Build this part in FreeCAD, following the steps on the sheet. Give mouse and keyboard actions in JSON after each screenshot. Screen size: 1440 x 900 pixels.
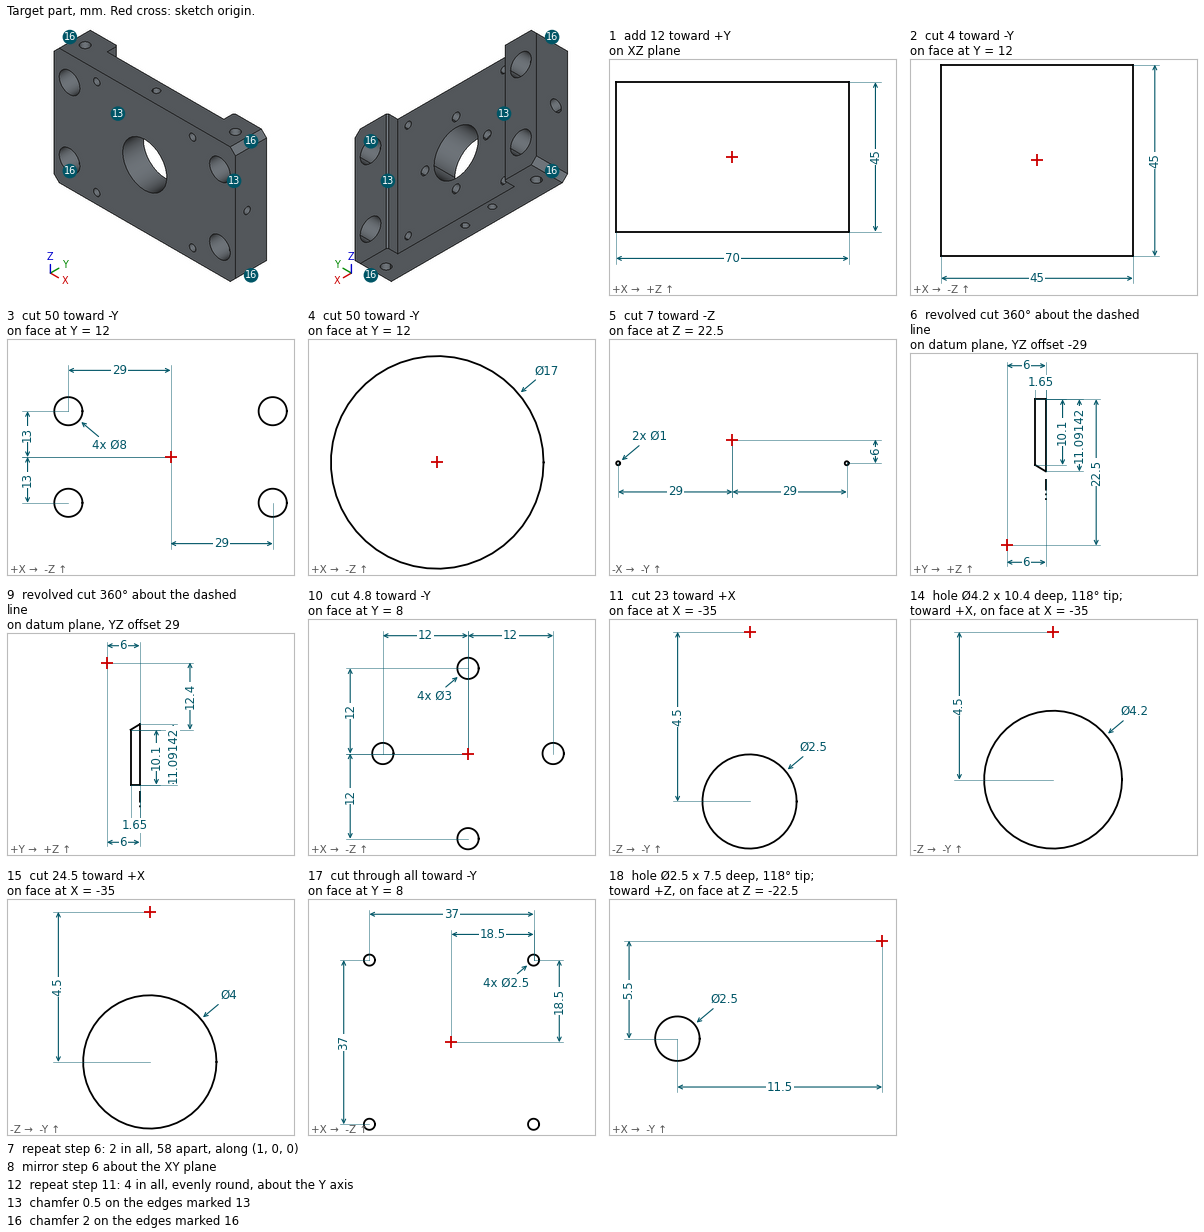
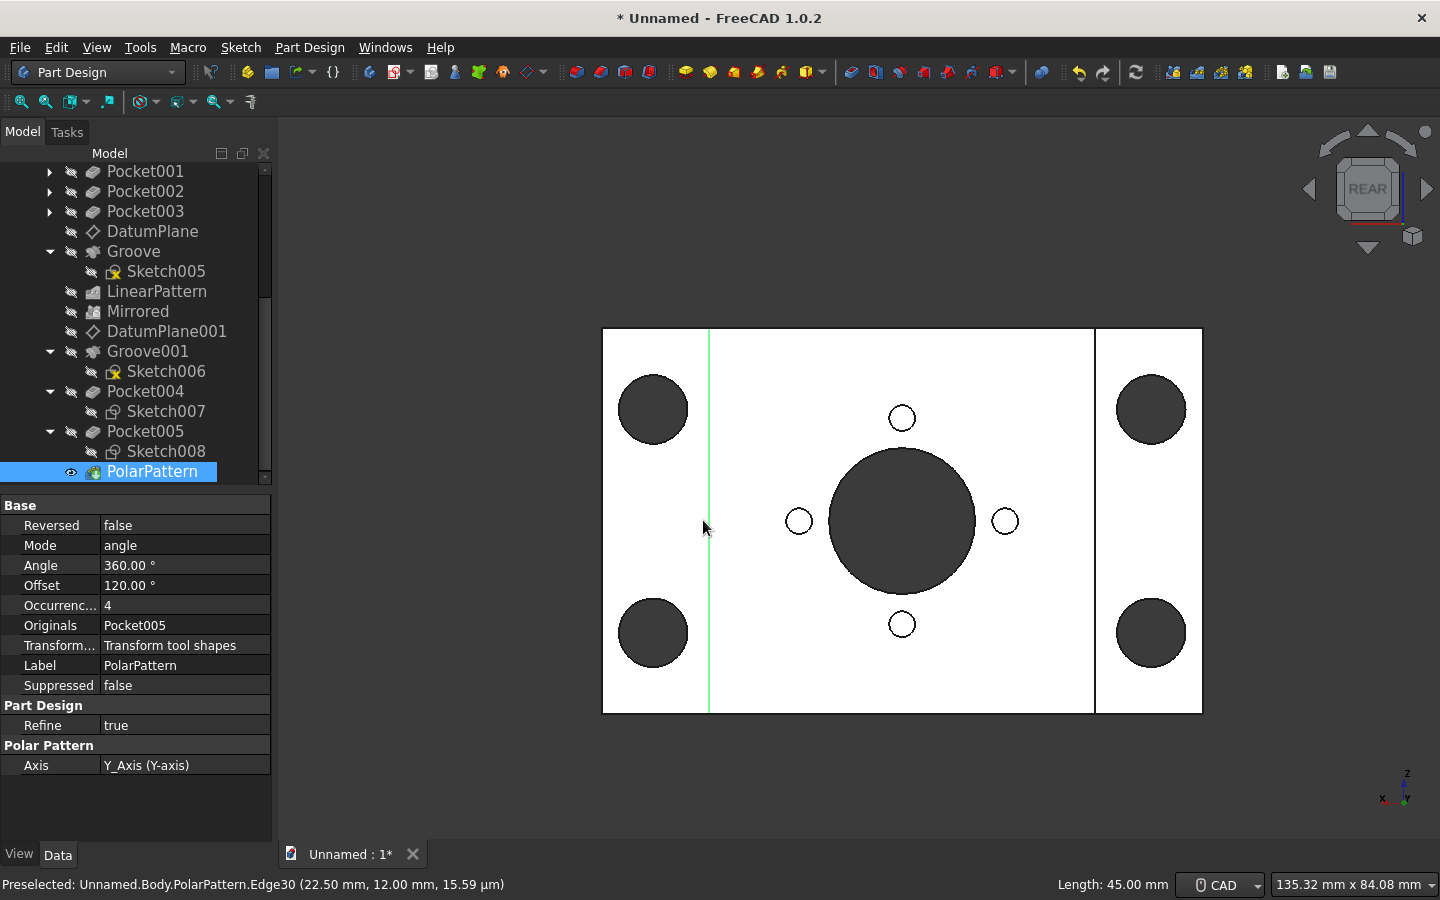
{"action": "left_click", "coordinate": [1095, 520], "text": "ctrl"}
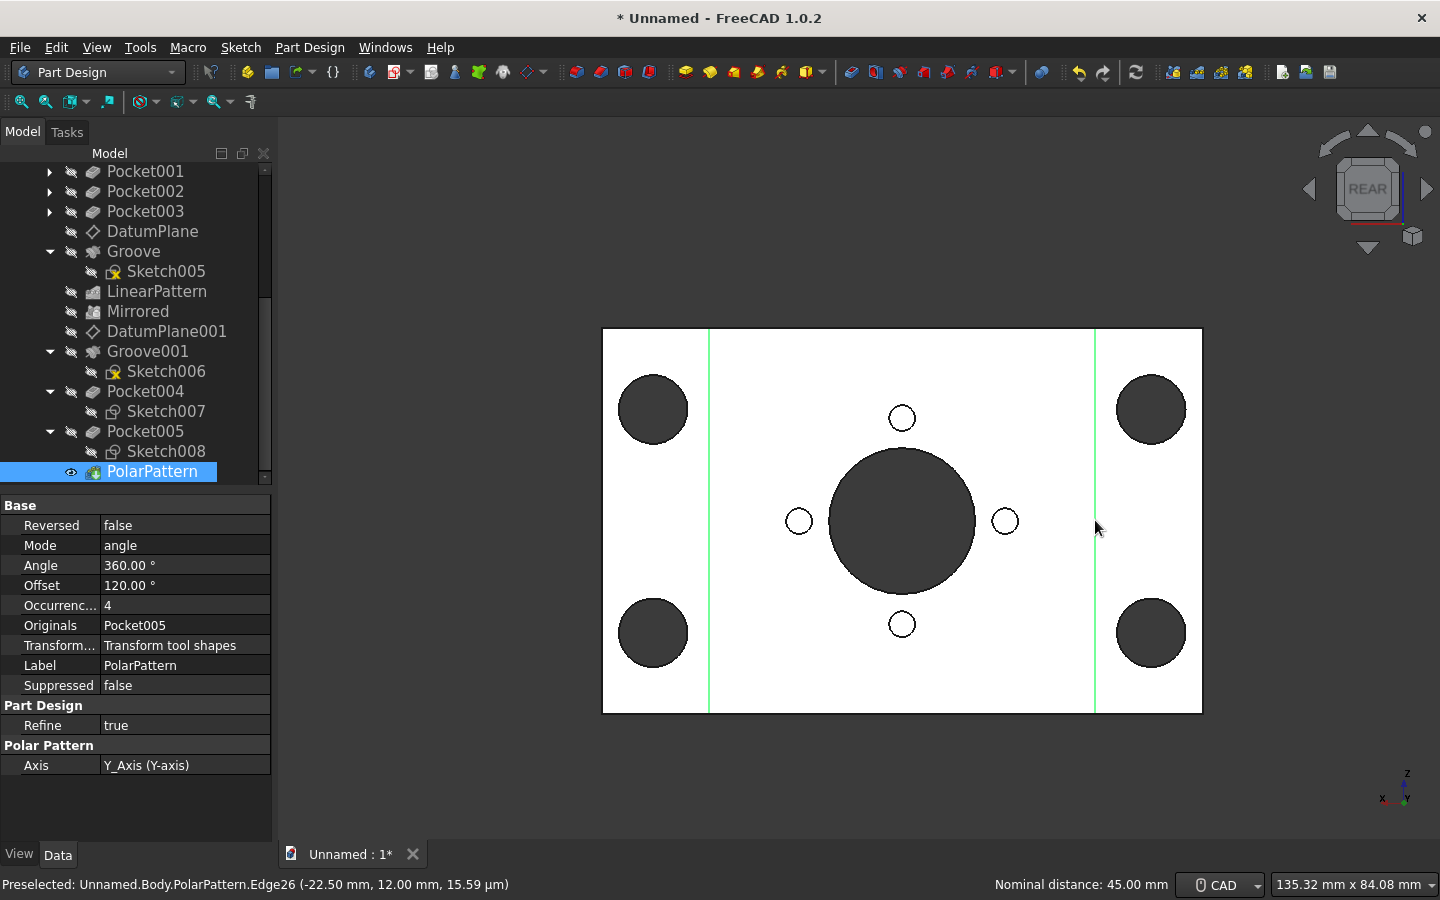
{"action": "left_click", "coordinate": [602, 72]}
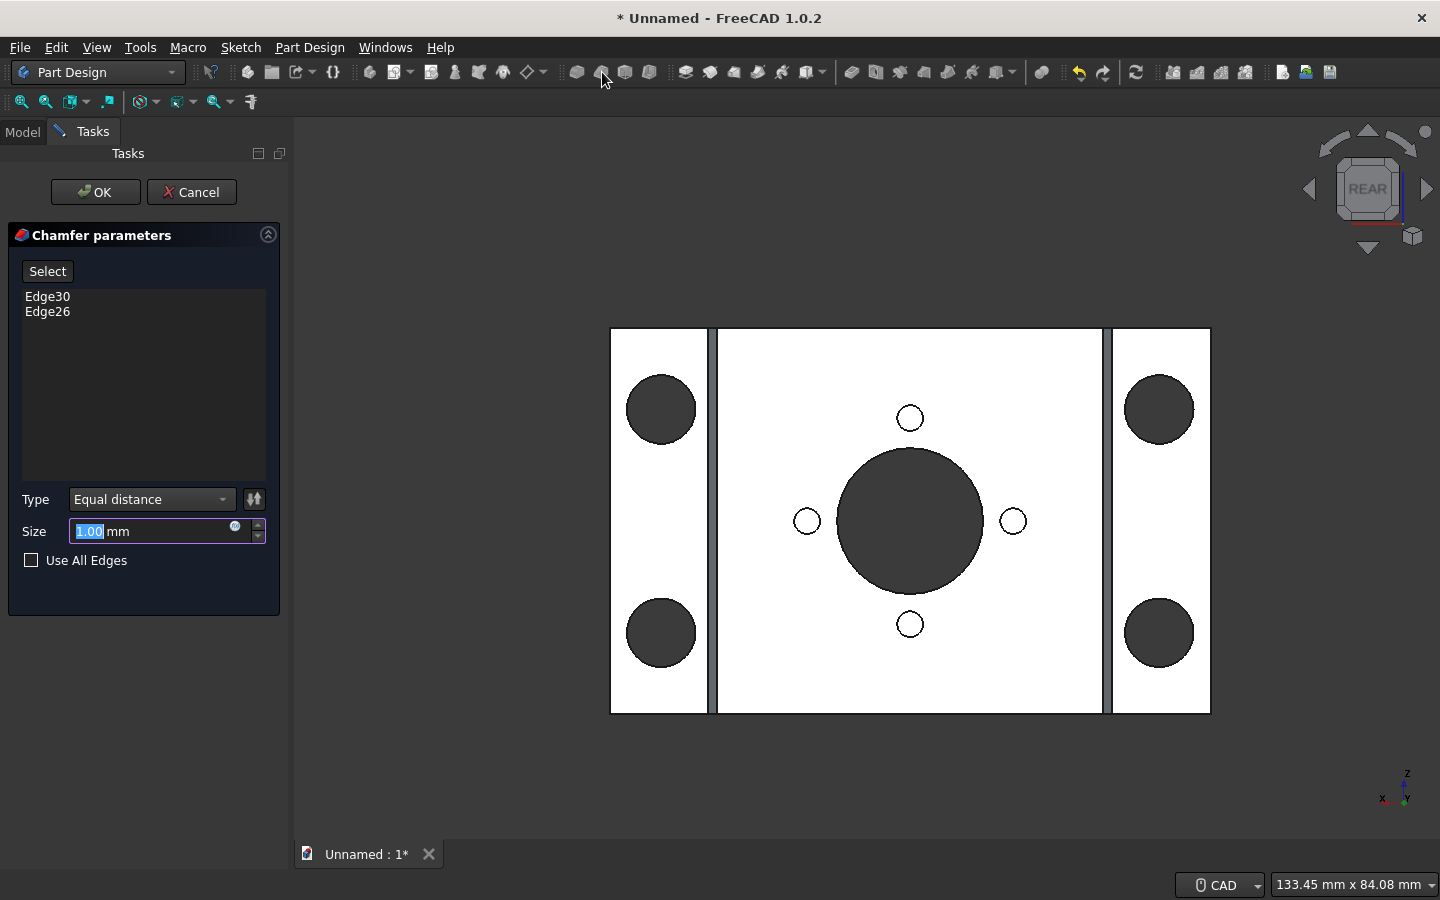
{"action": "type", "text": "0.5"}
{"action": "key", "text": "Tab"}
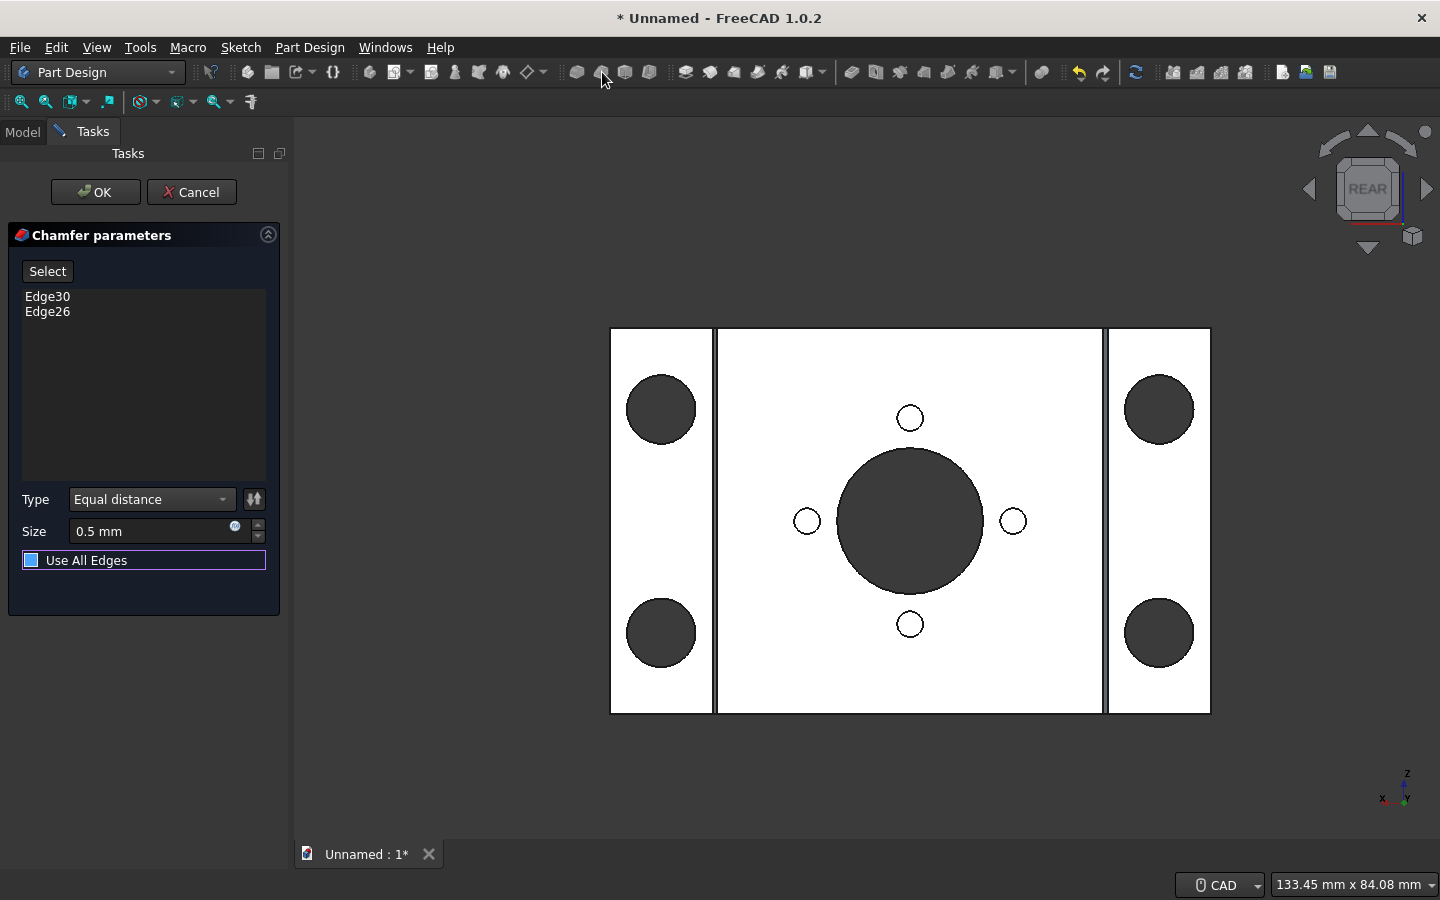
{"action": "left_click", "coordinate": [96, 192]}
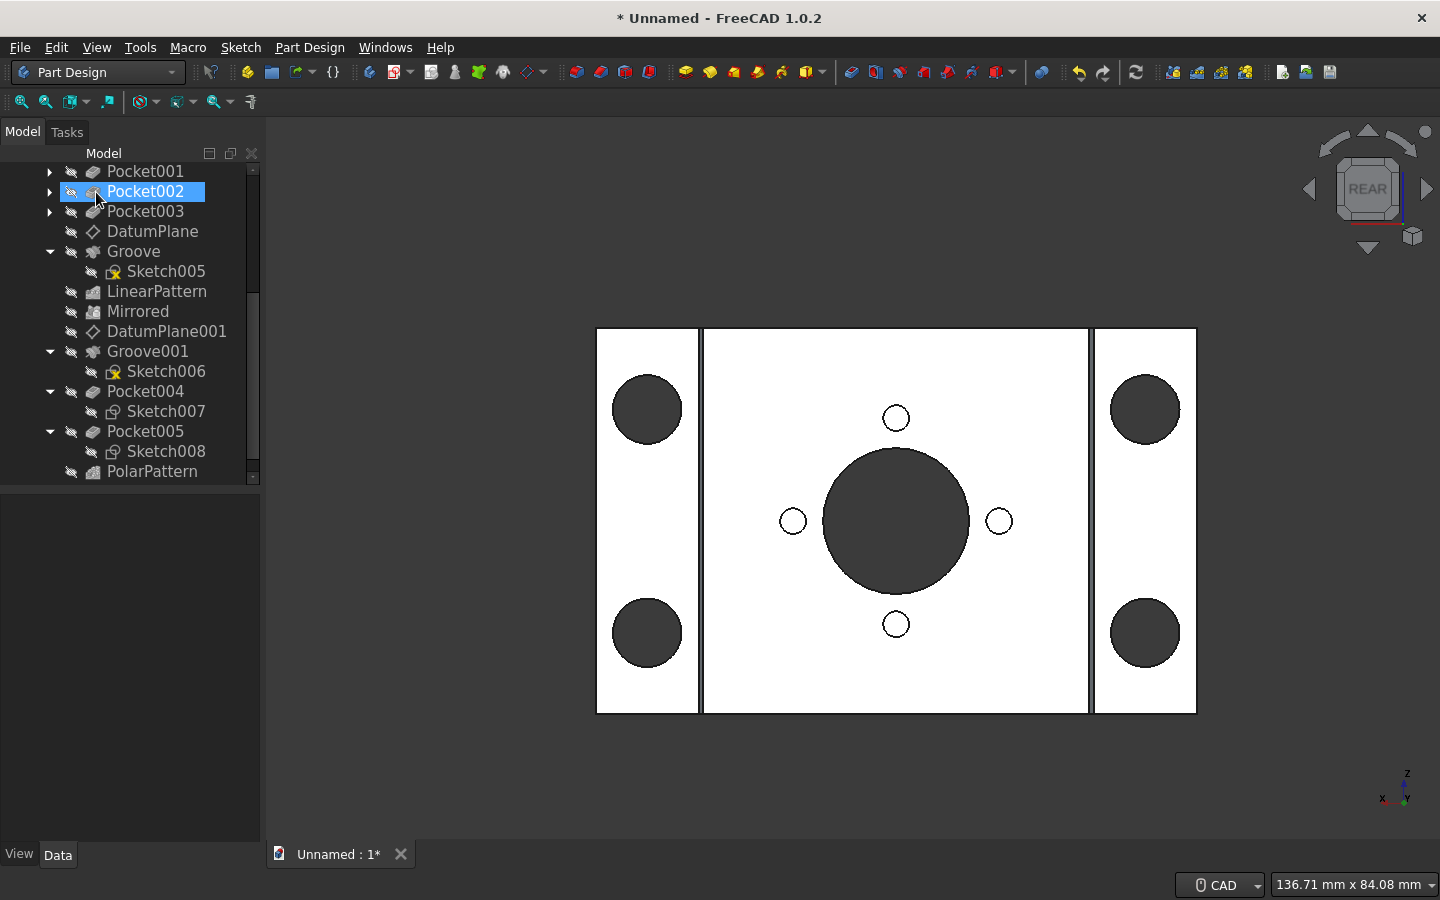
{"action": "key", "text": "6"}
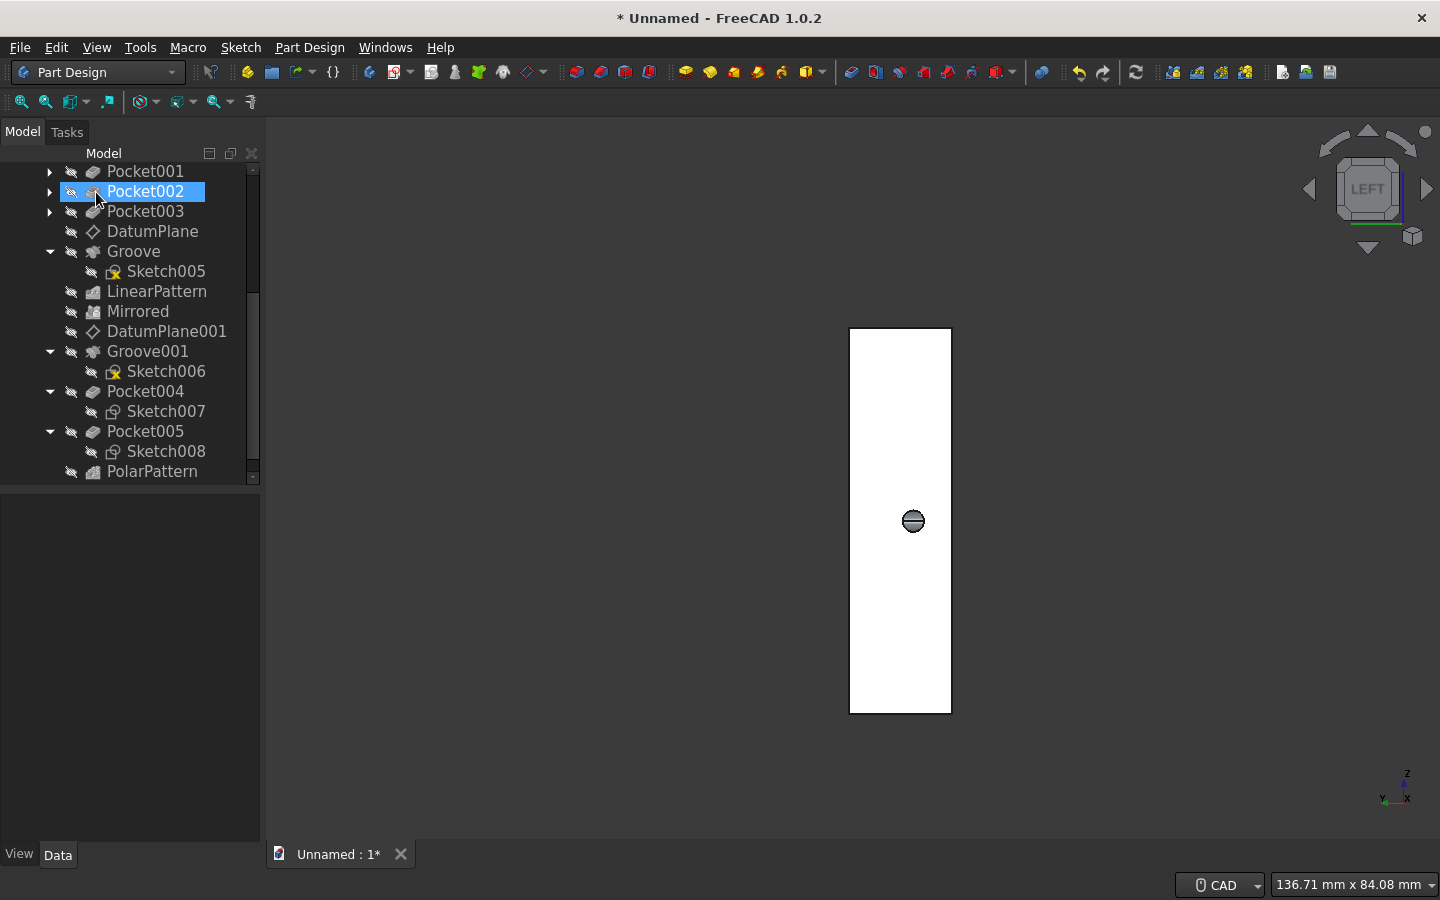
{"action": "left_click", "coordinate": [900, 410]}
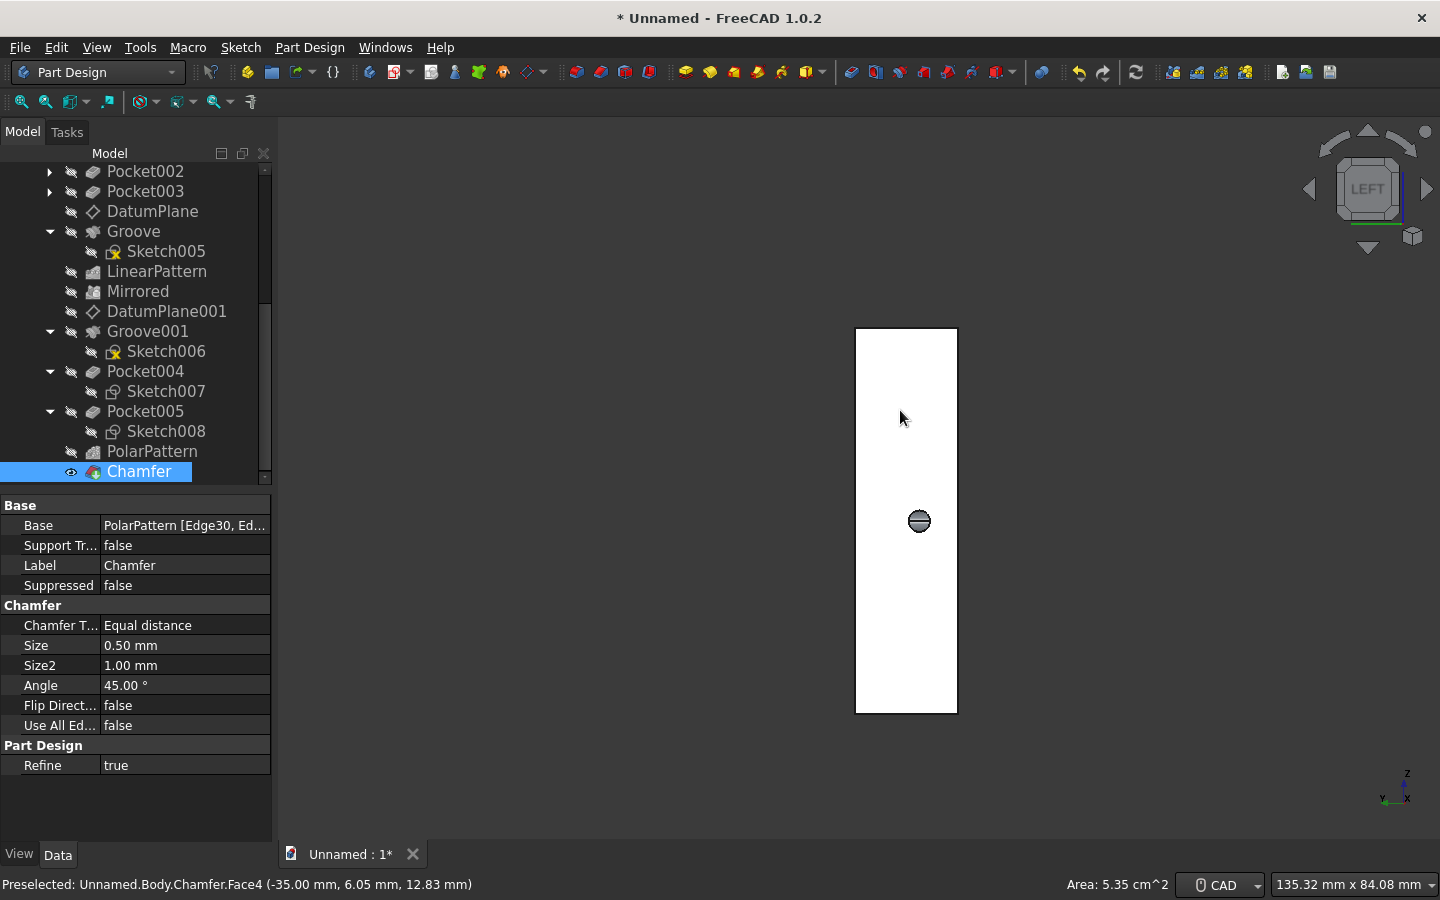
{"action": "left_click", "coordinate": [394, 72]}